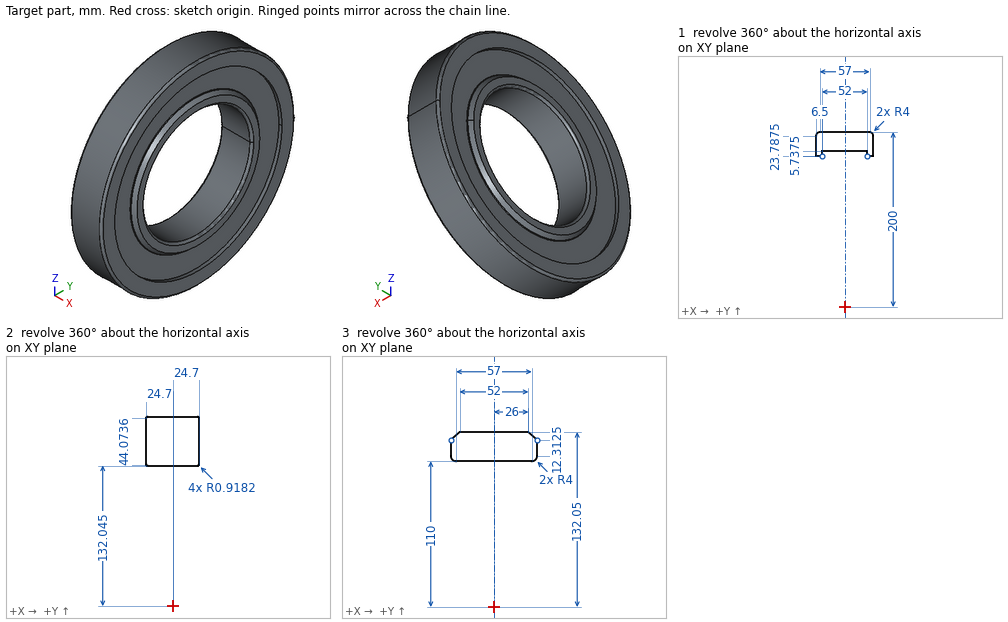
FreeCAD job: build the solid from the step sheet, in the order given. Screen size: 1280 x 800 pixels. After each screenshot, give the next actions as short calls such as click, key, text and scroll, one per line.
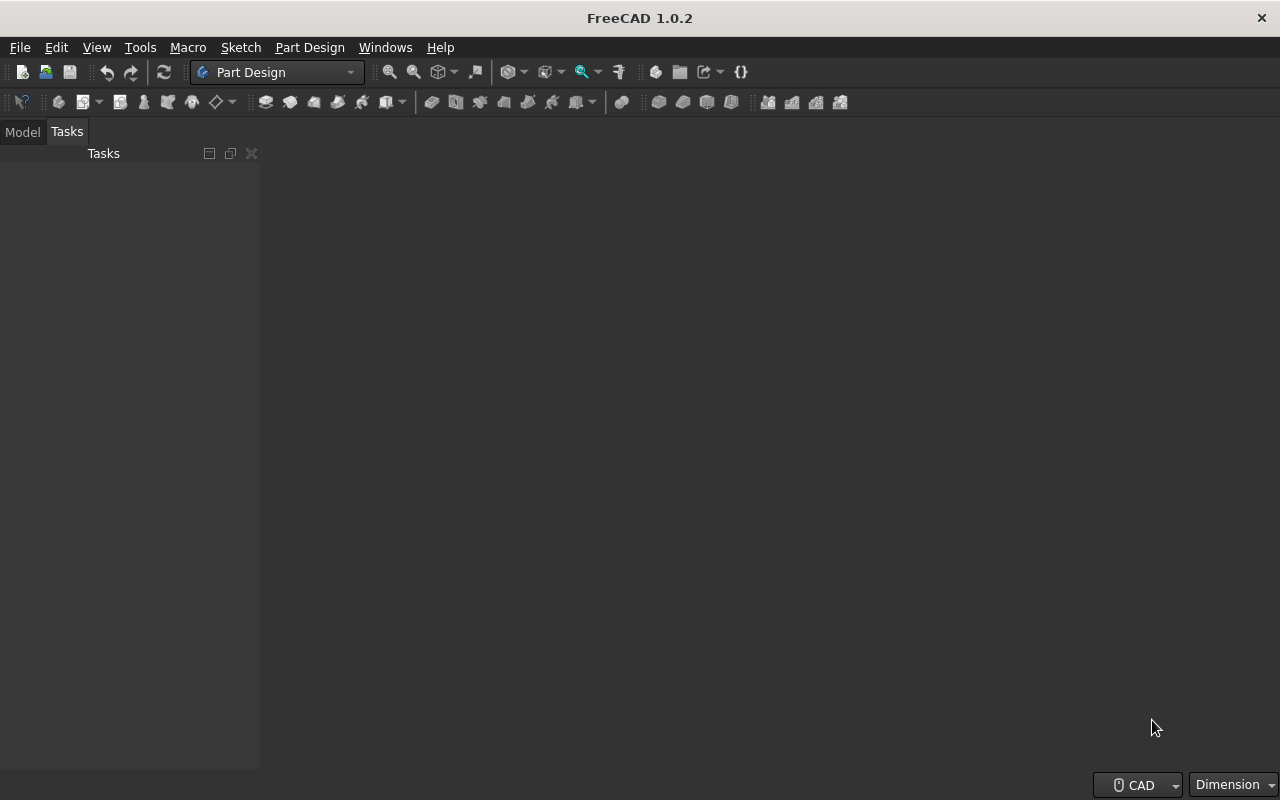
click(290, 72)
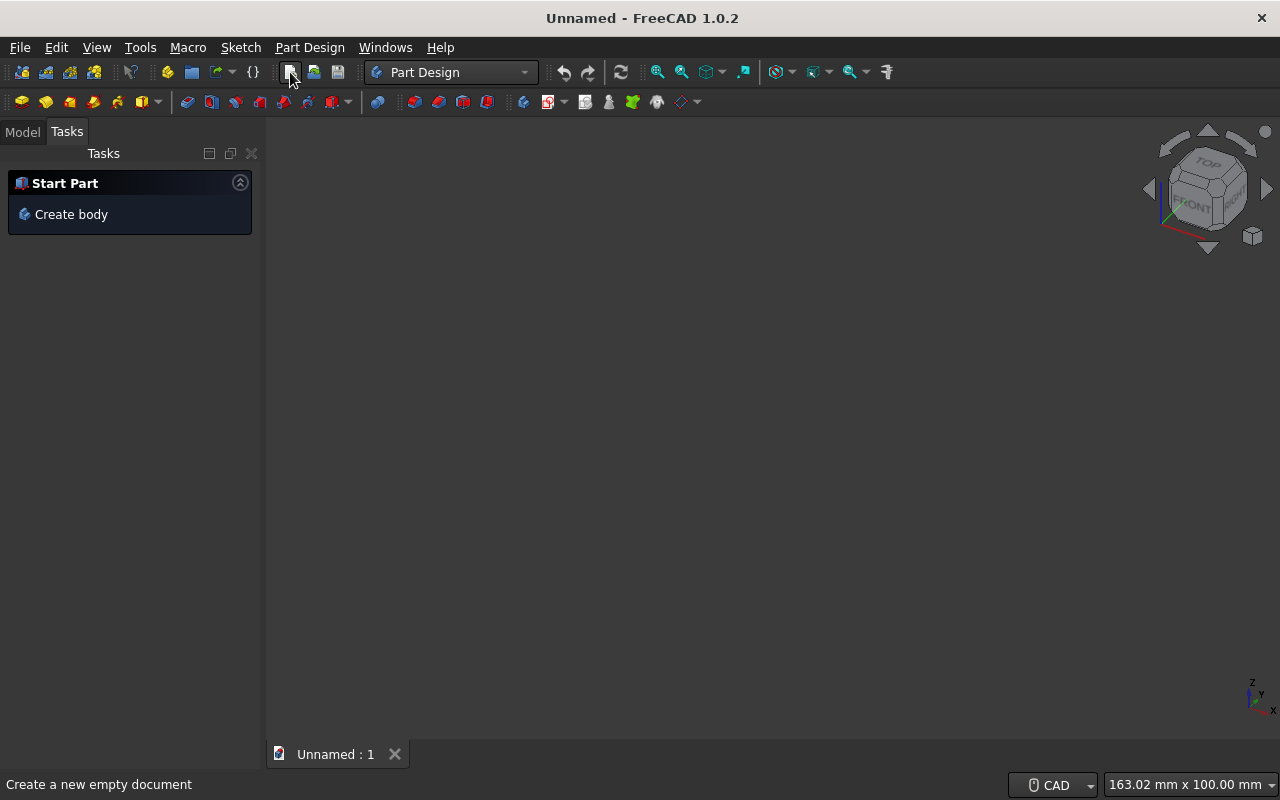
click(548, 102)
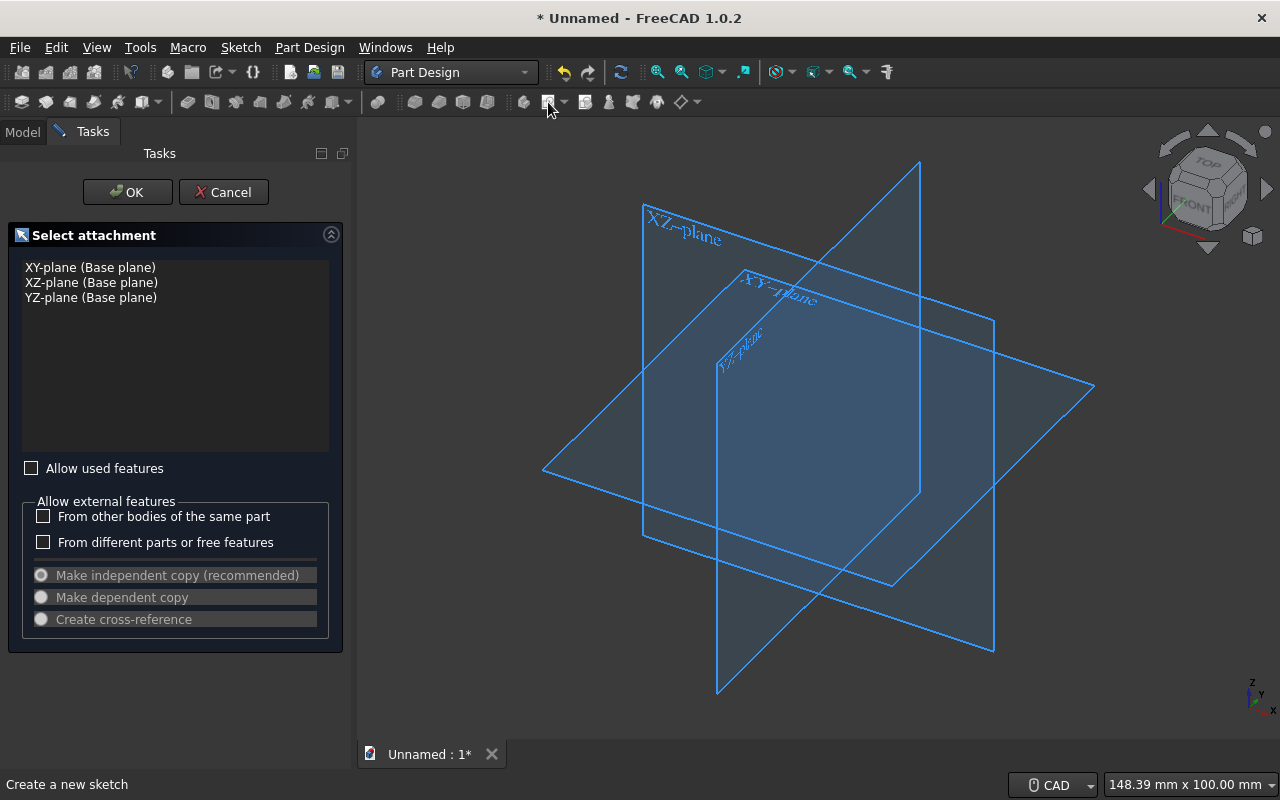
click(82, 268)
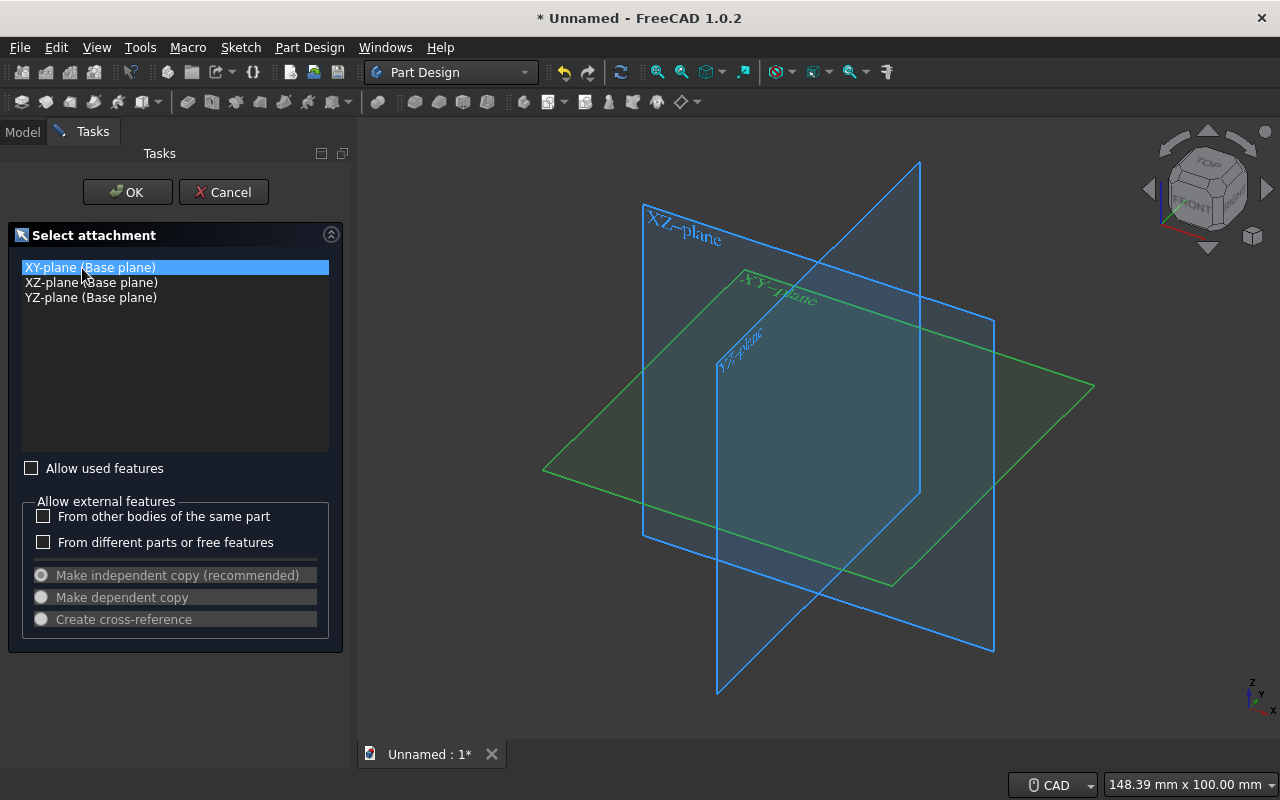
click(128, 192)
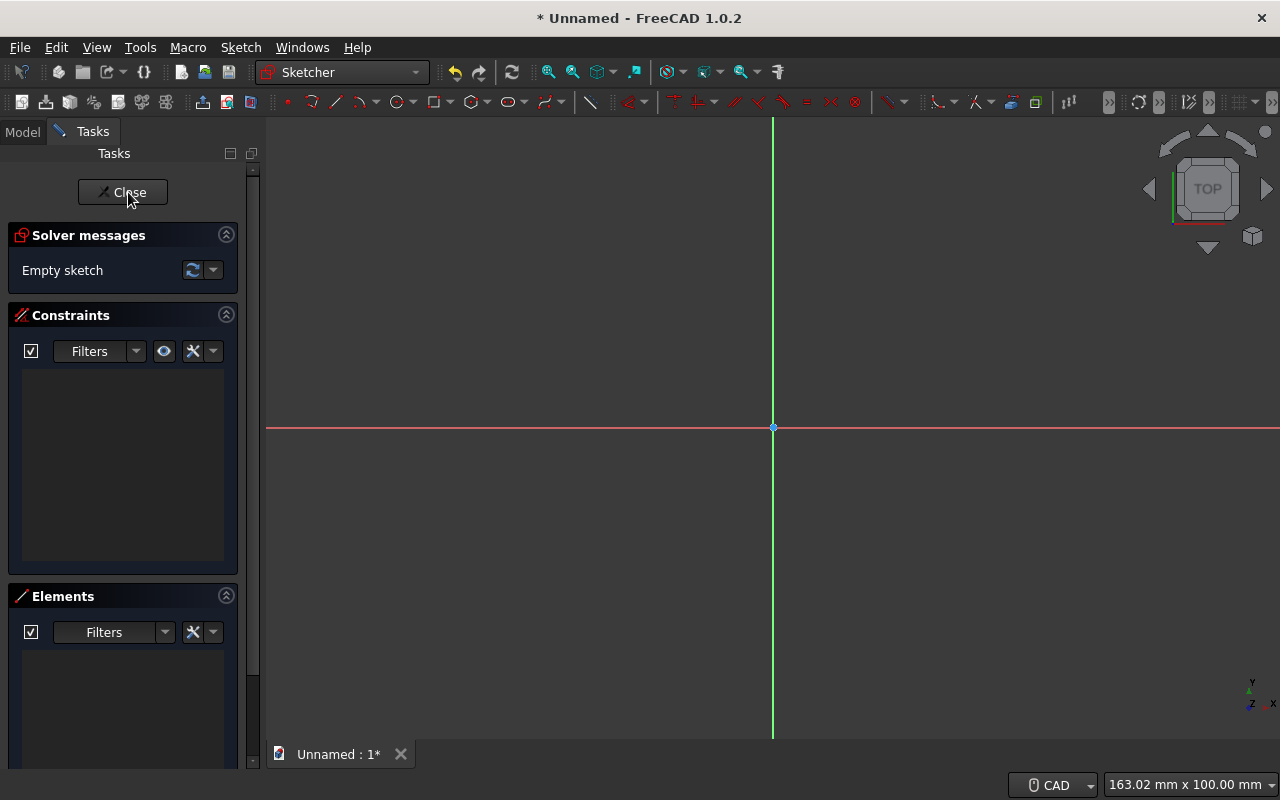
scroll(704, 428, down, 5)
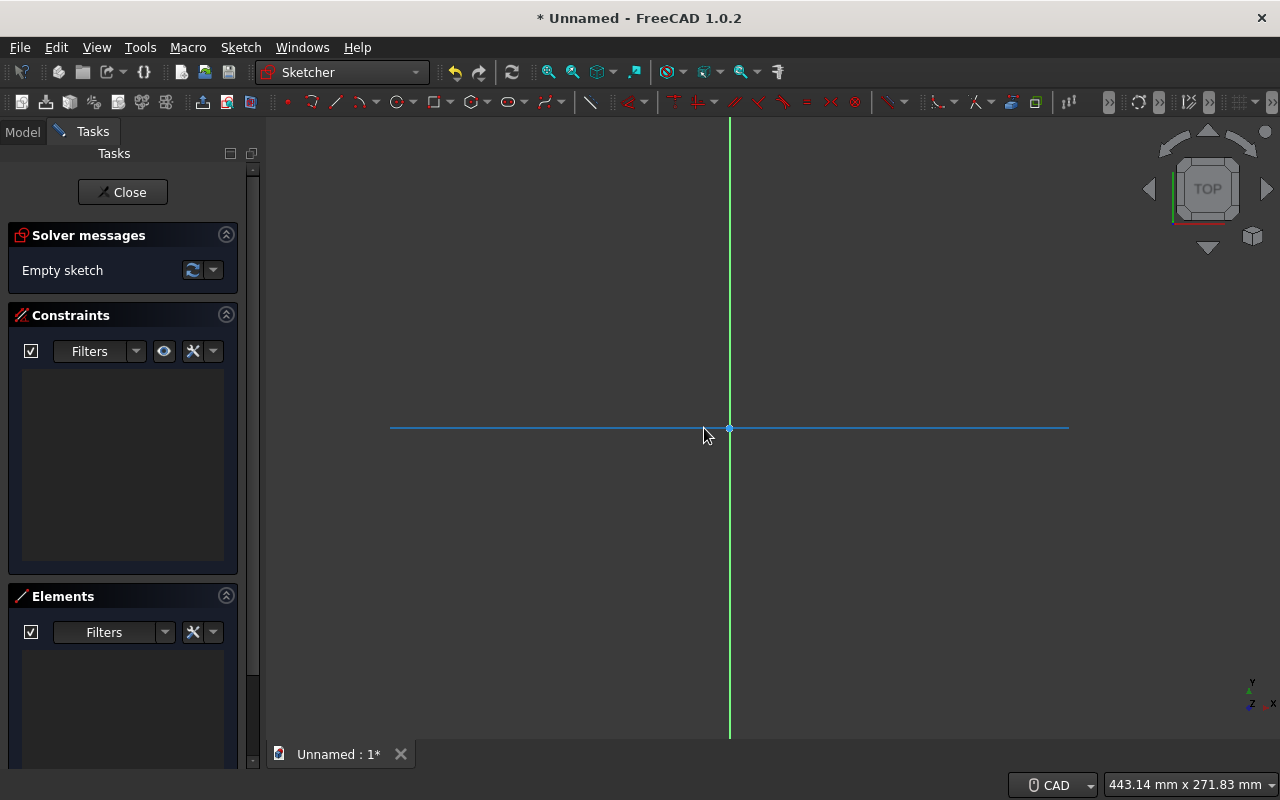
scroll(704, 428, down, 5)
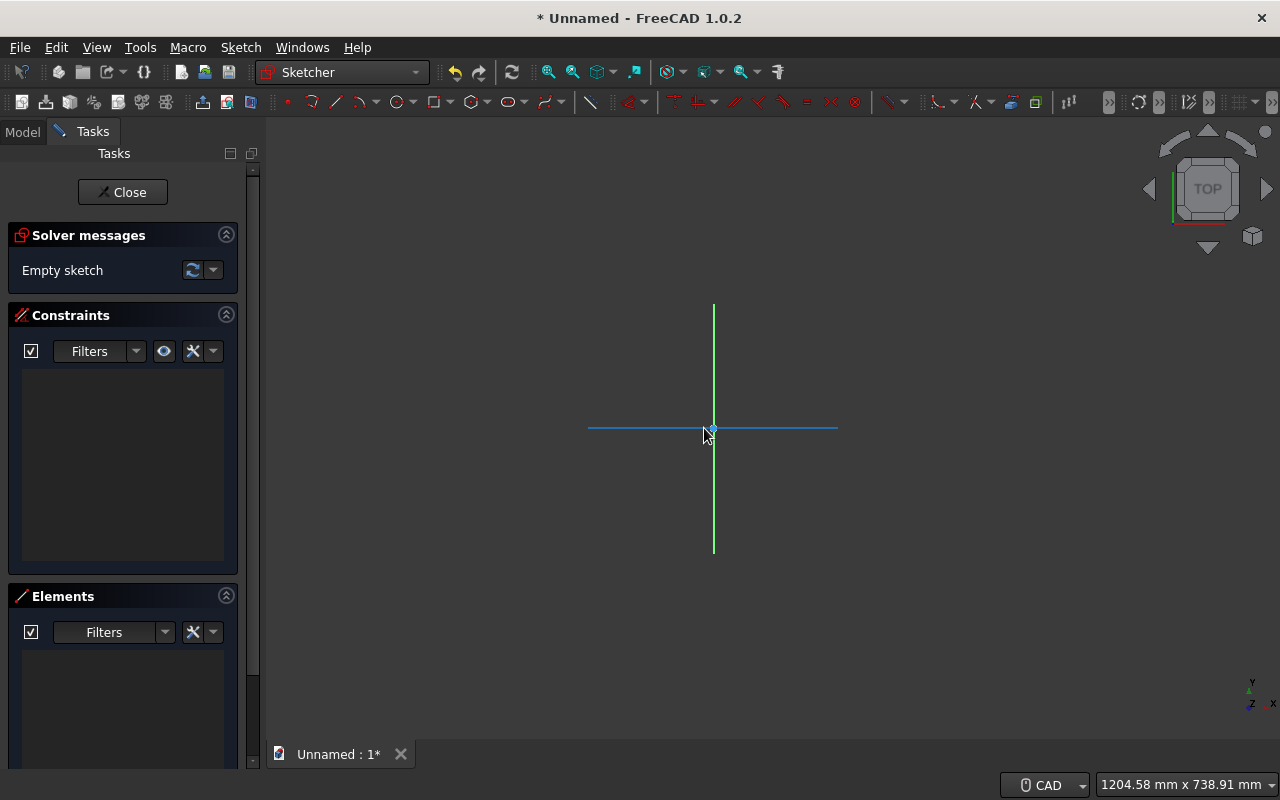
scroll(715, 256, up, 12)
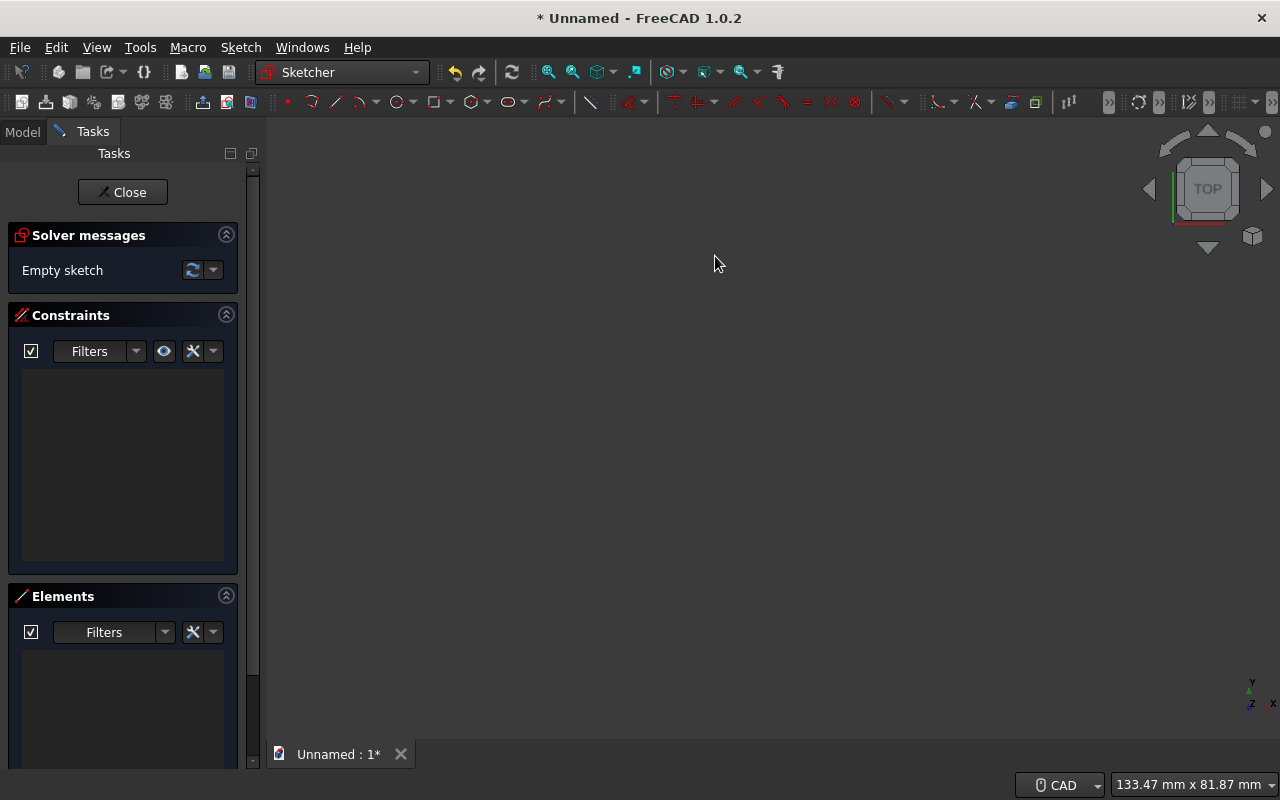
click(336, 102)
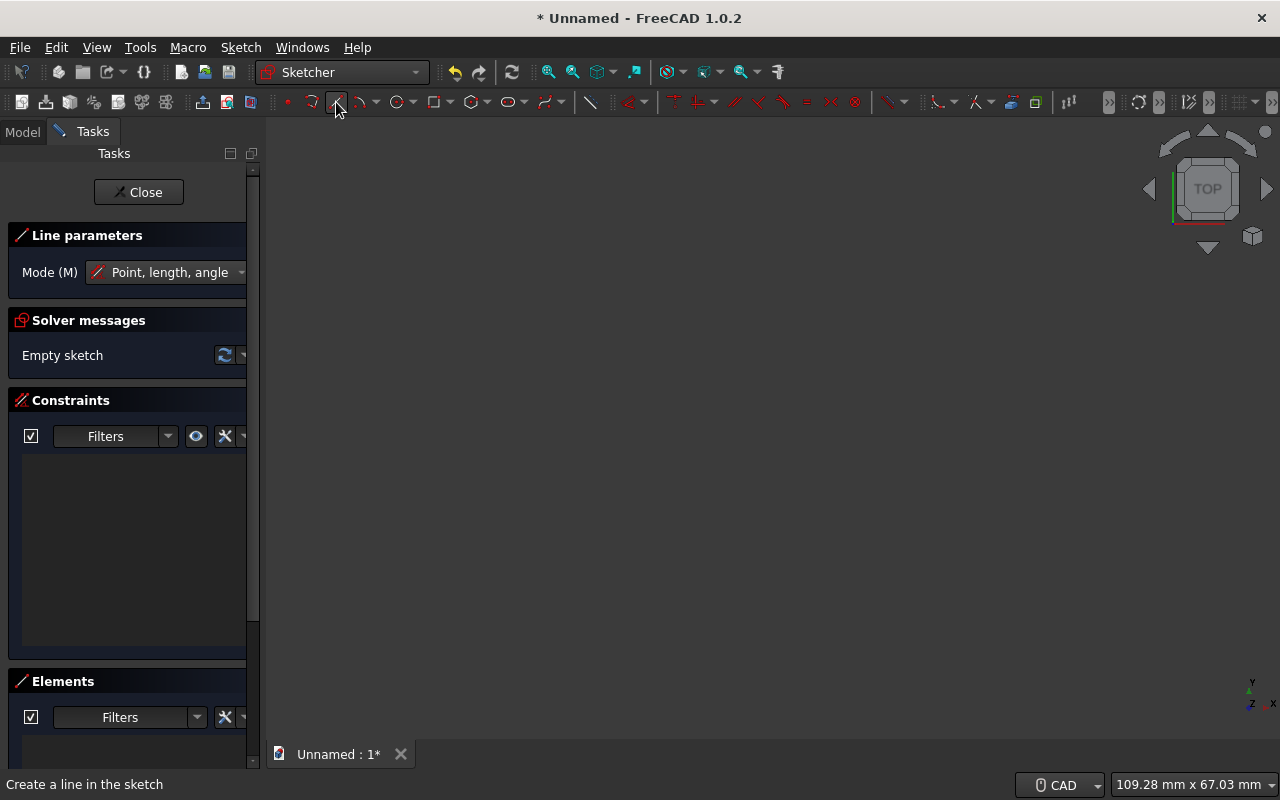
click(961, 299)
click(432, 299)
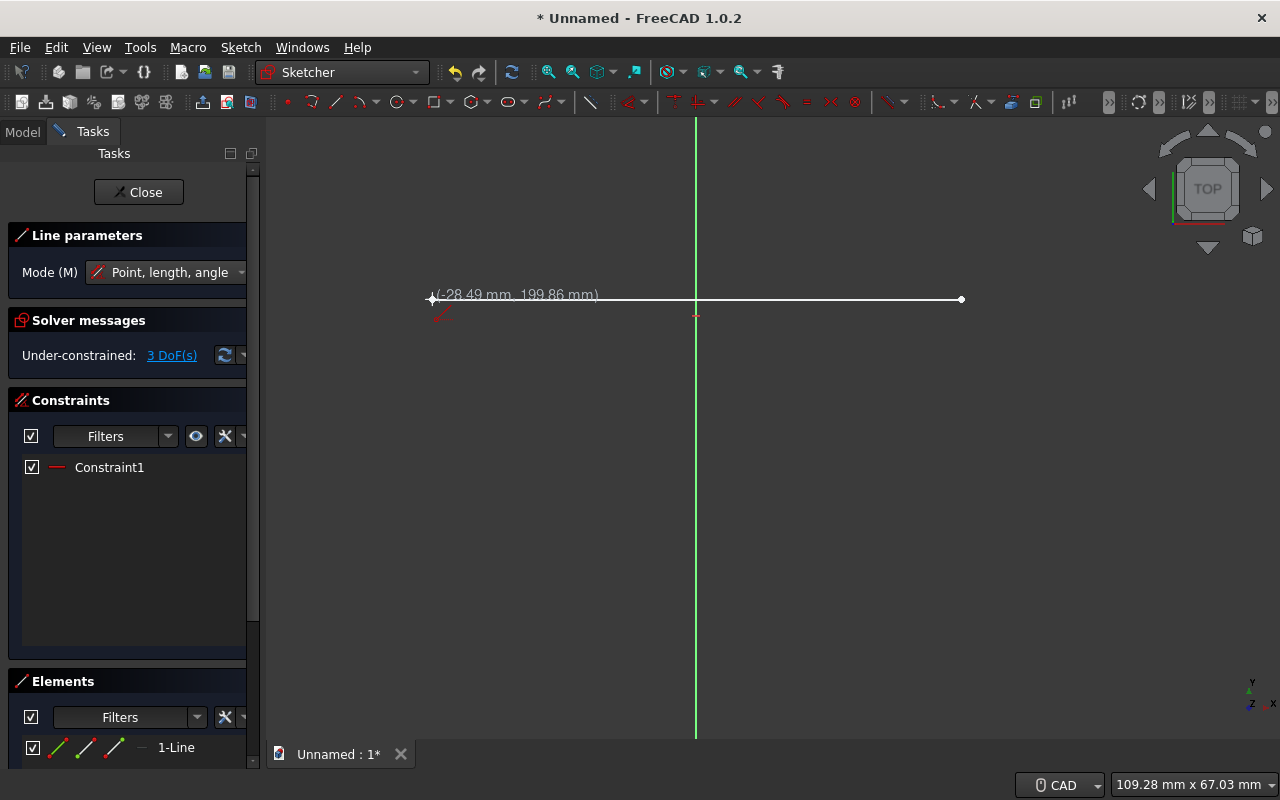
click(312, 102)